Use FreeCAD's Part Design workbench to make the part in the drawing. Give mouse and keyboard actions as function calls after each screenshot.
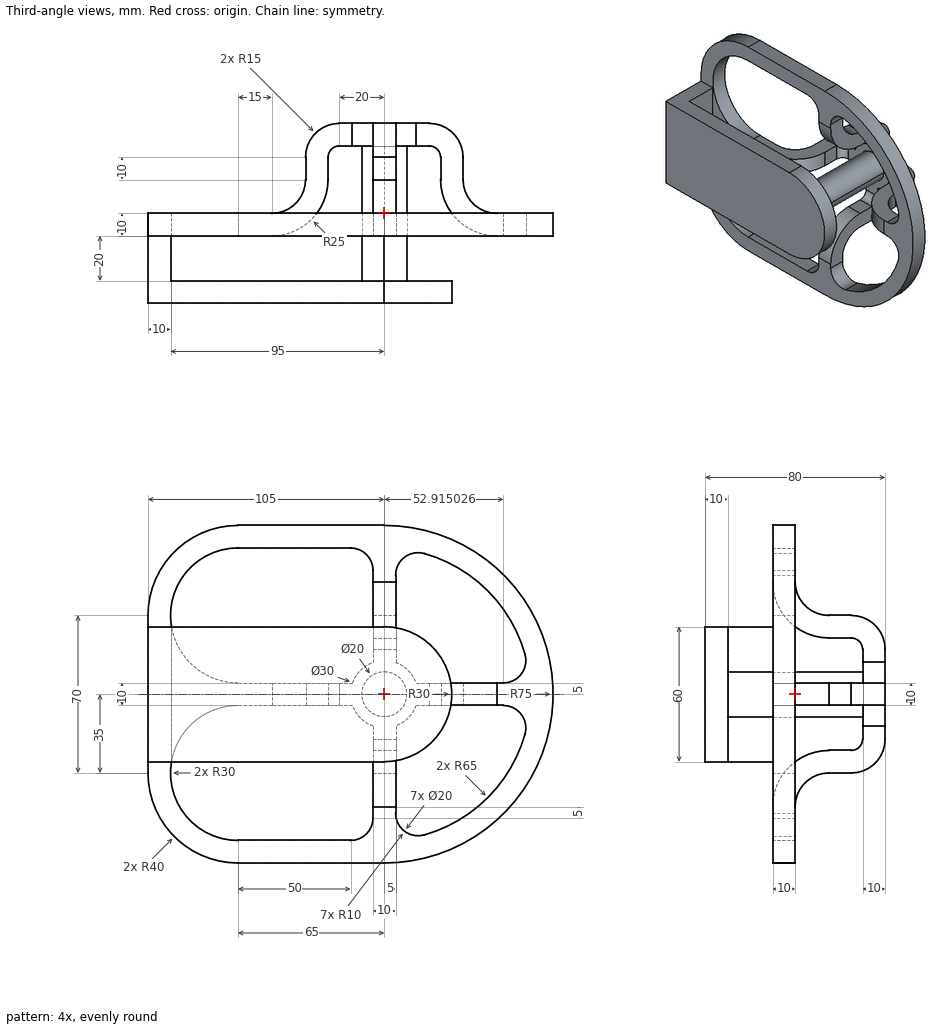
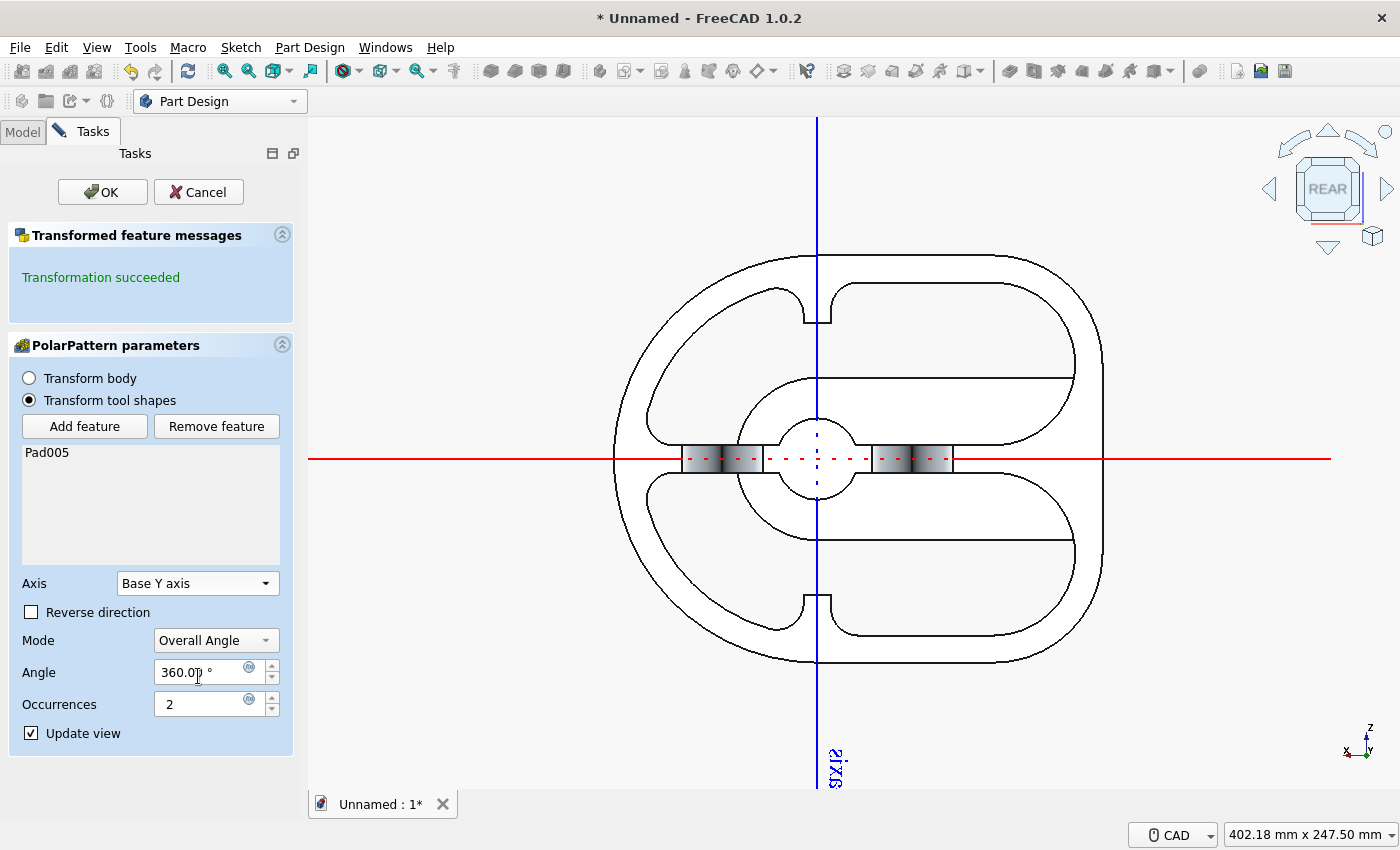
triple_click(209, 704)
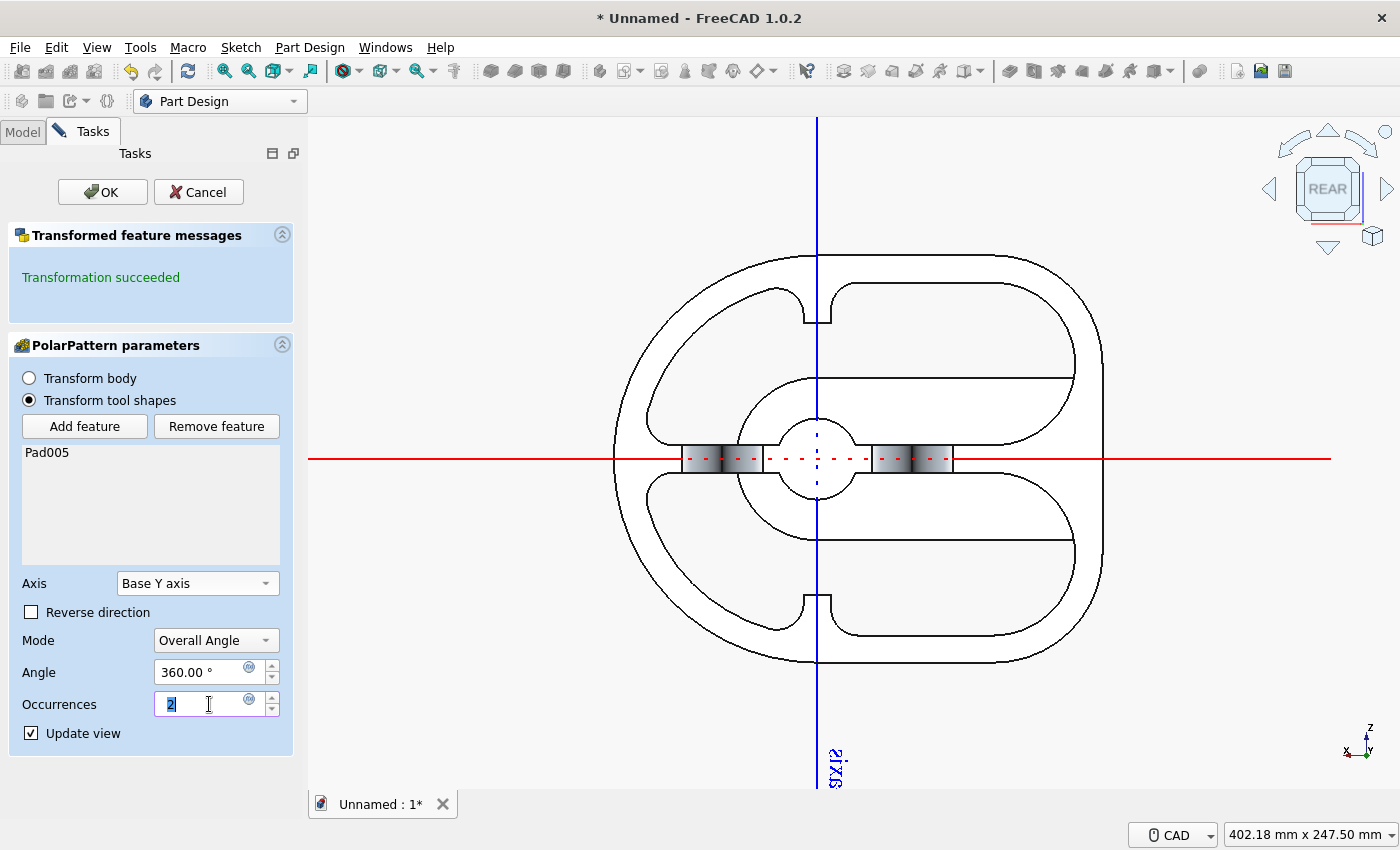
text(4)
key(Tab)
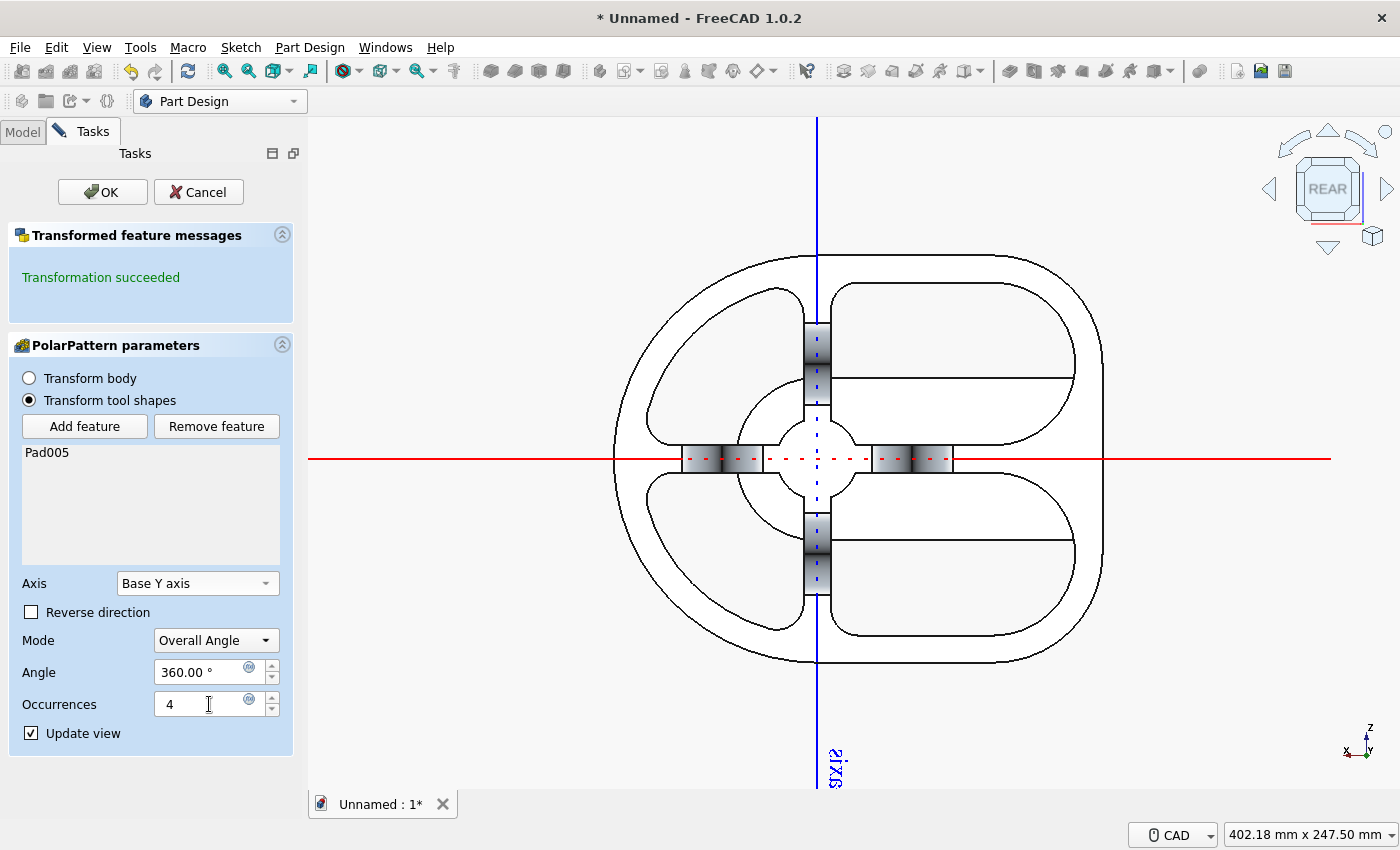
click(103, 192)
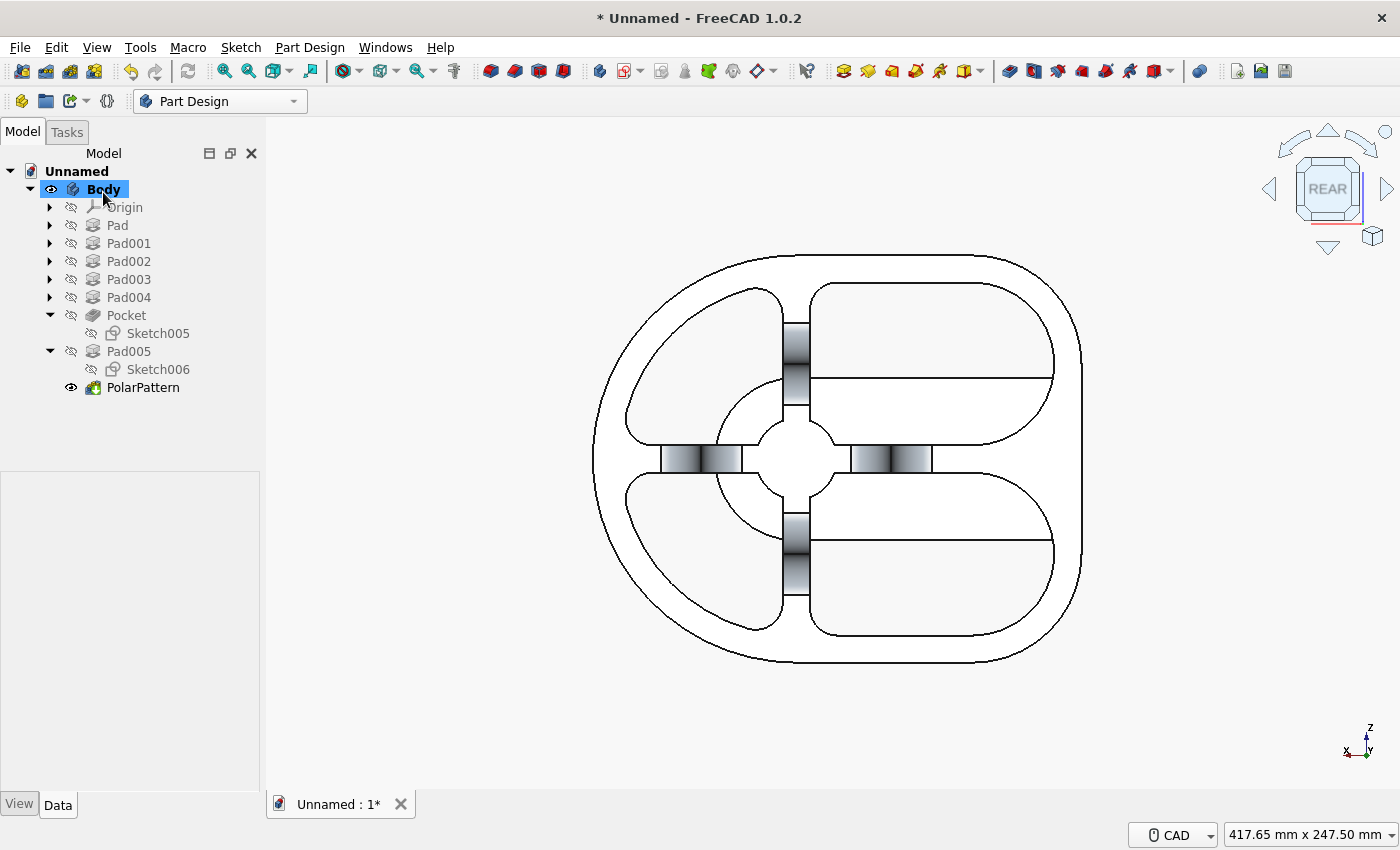
key(0)